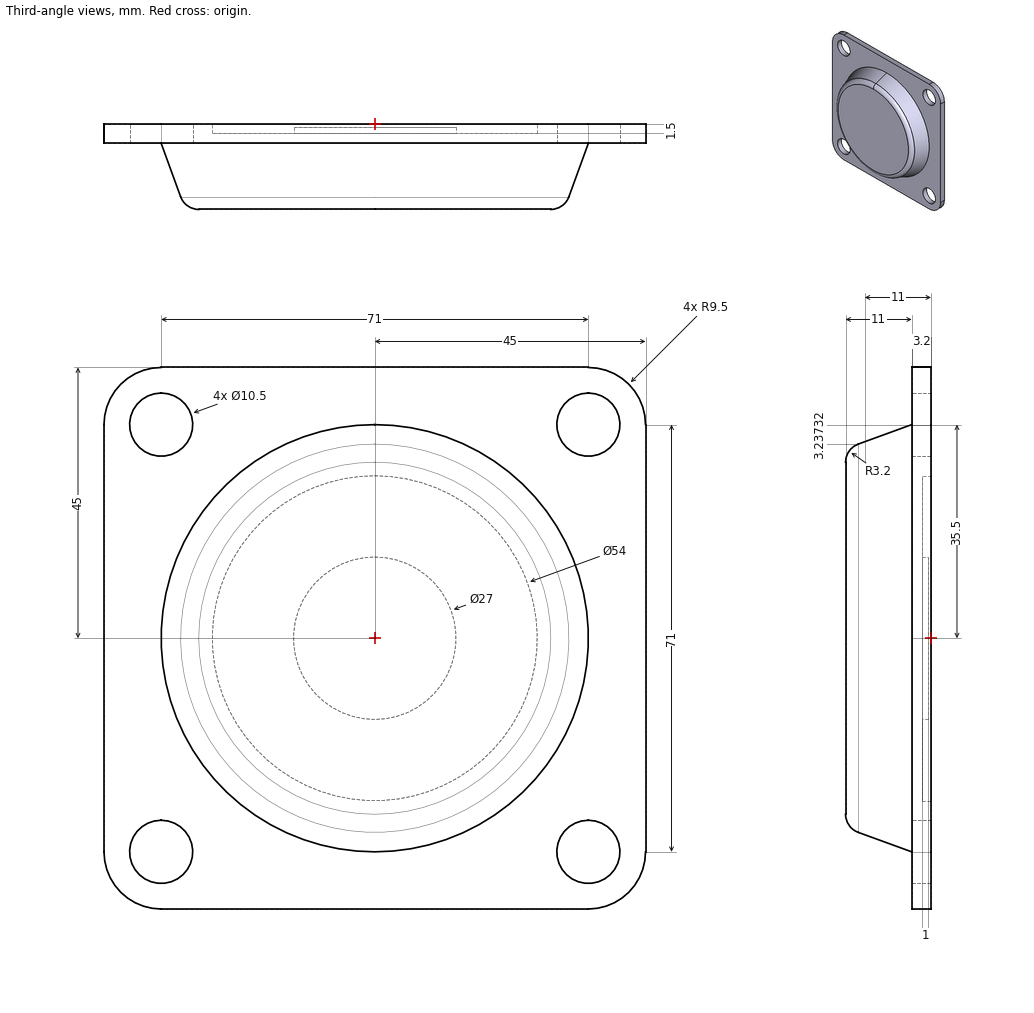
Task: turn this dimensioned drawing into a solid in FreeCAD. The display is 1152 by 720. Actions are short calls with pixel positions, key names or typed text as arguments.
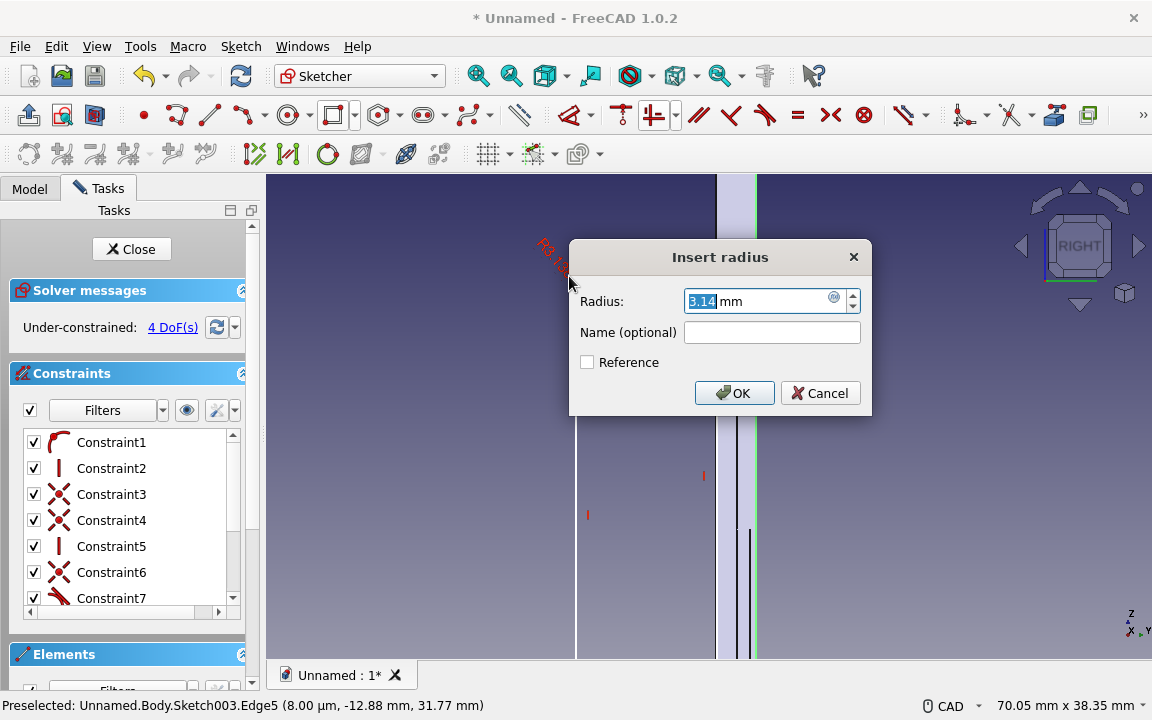
text(3.2)
key(Return)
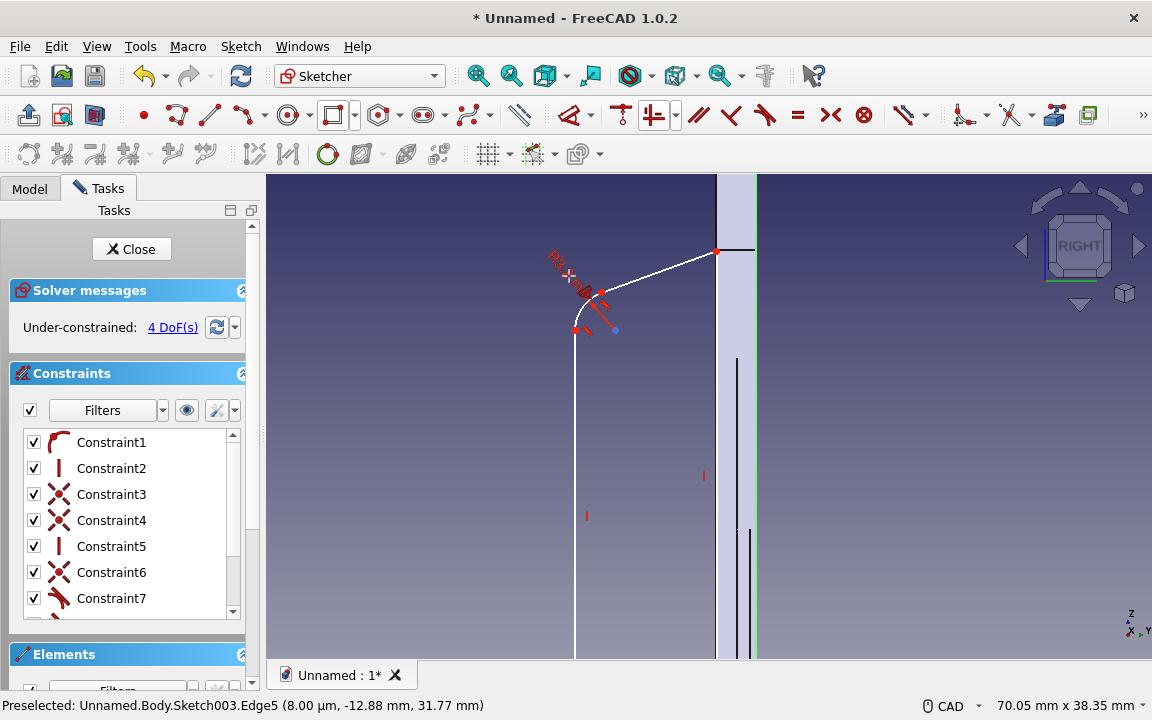
scroll(588, 298, down, 2)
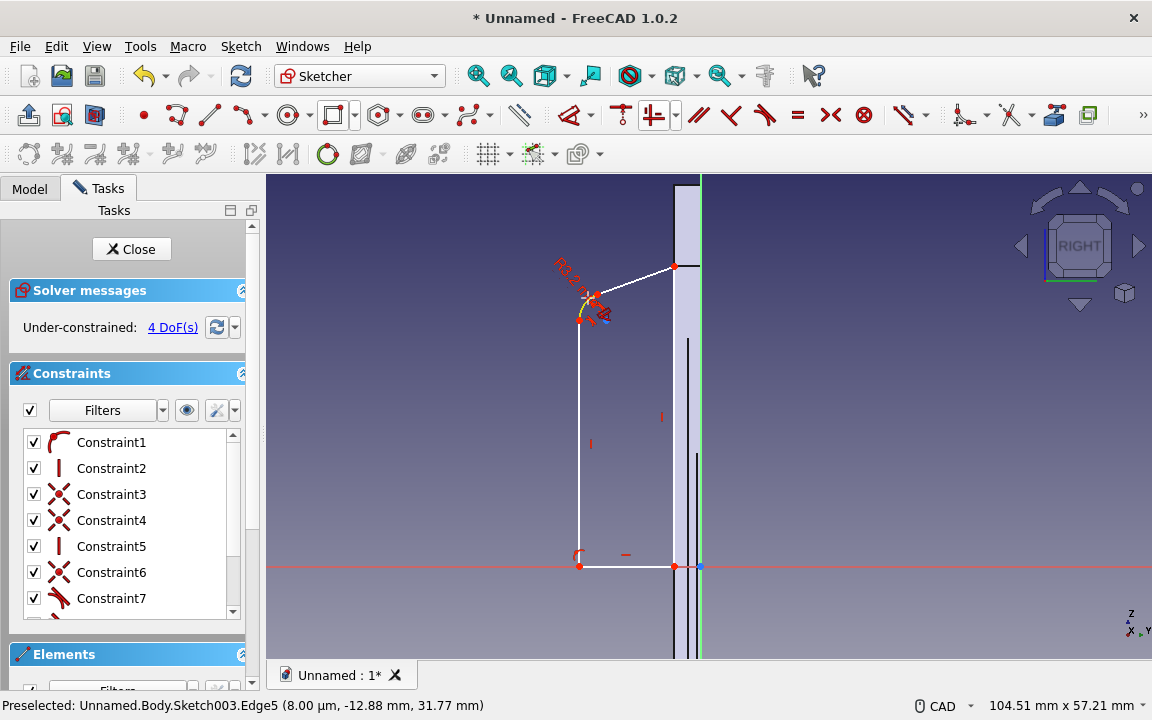
click(608, 567)
click(627, 601)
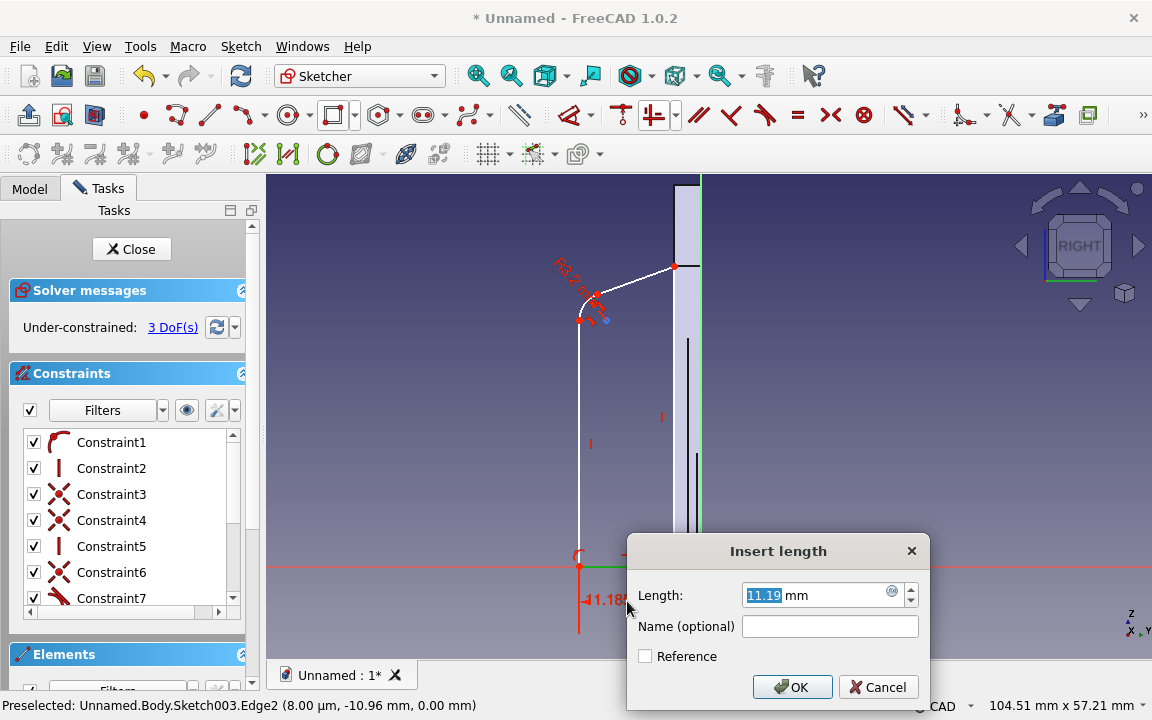
text(11)
key(Return)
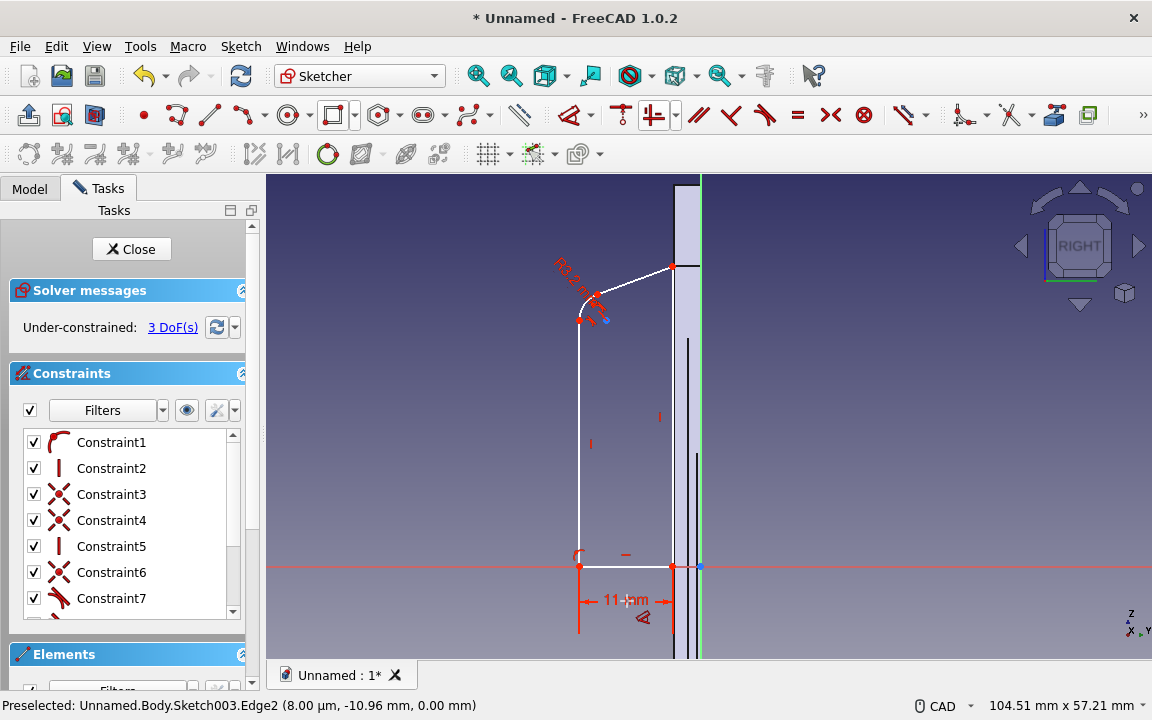
click(607, 320)
click(687, 286)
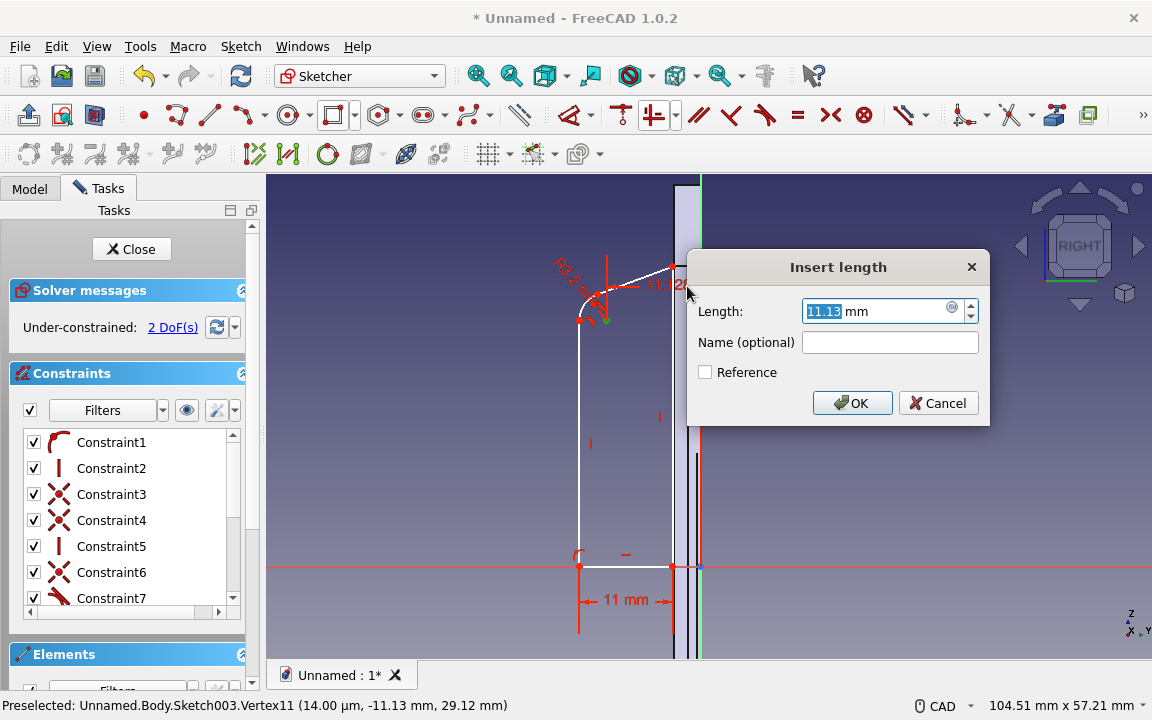
text(11)
key(Return)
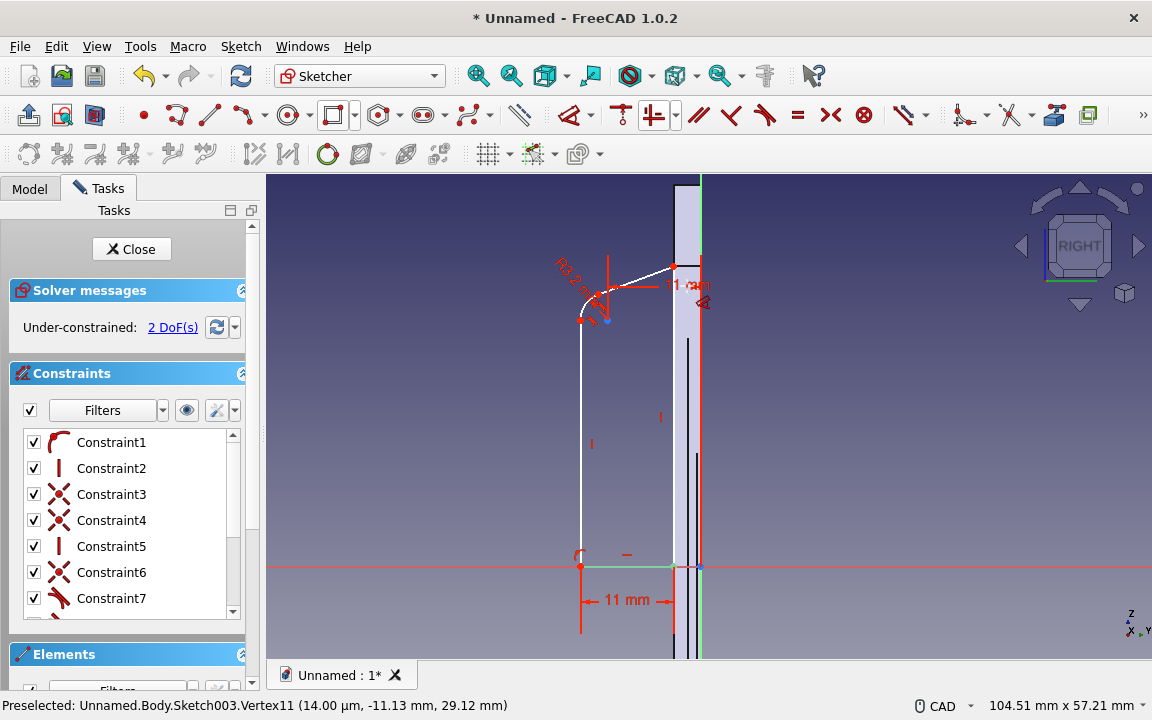
click(674, 477)
click(640, 417)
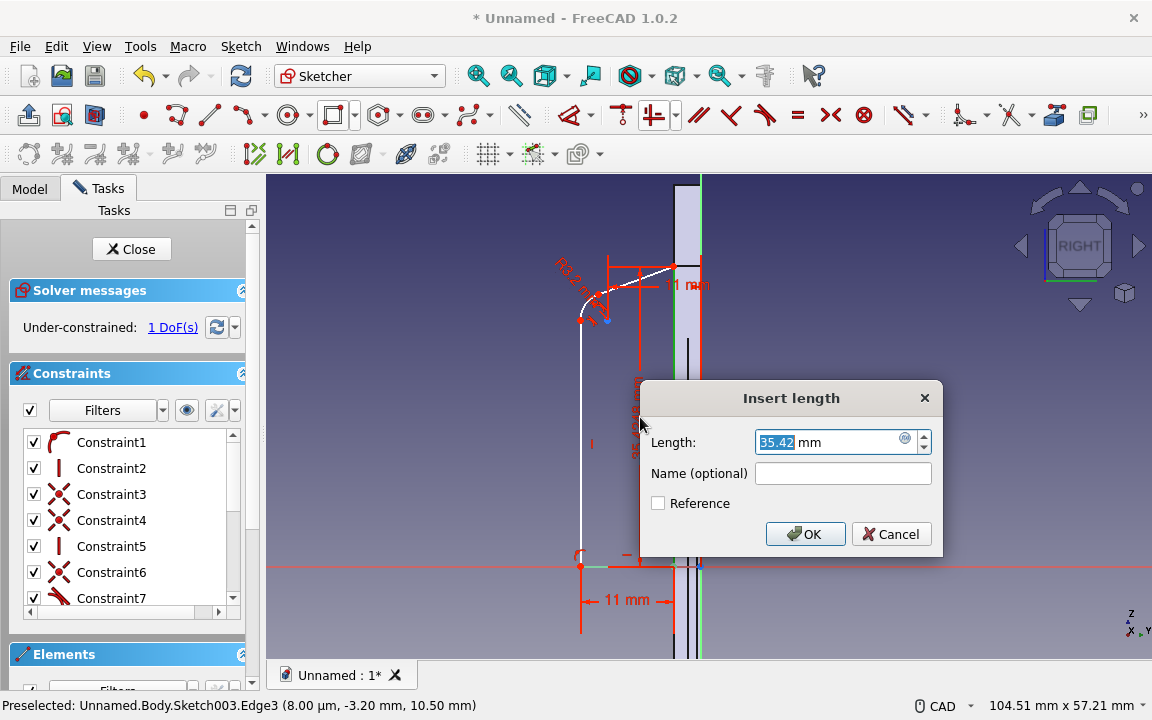
text(35.5)
key(Return)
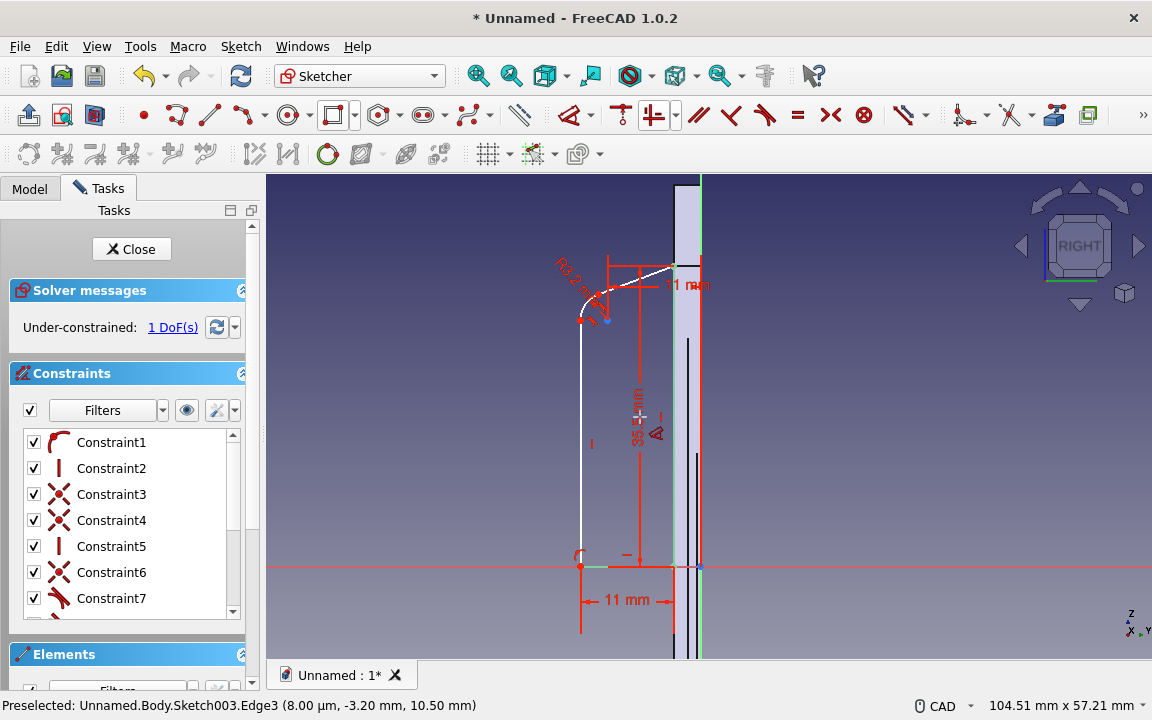
scroll(651, 275, up, 2)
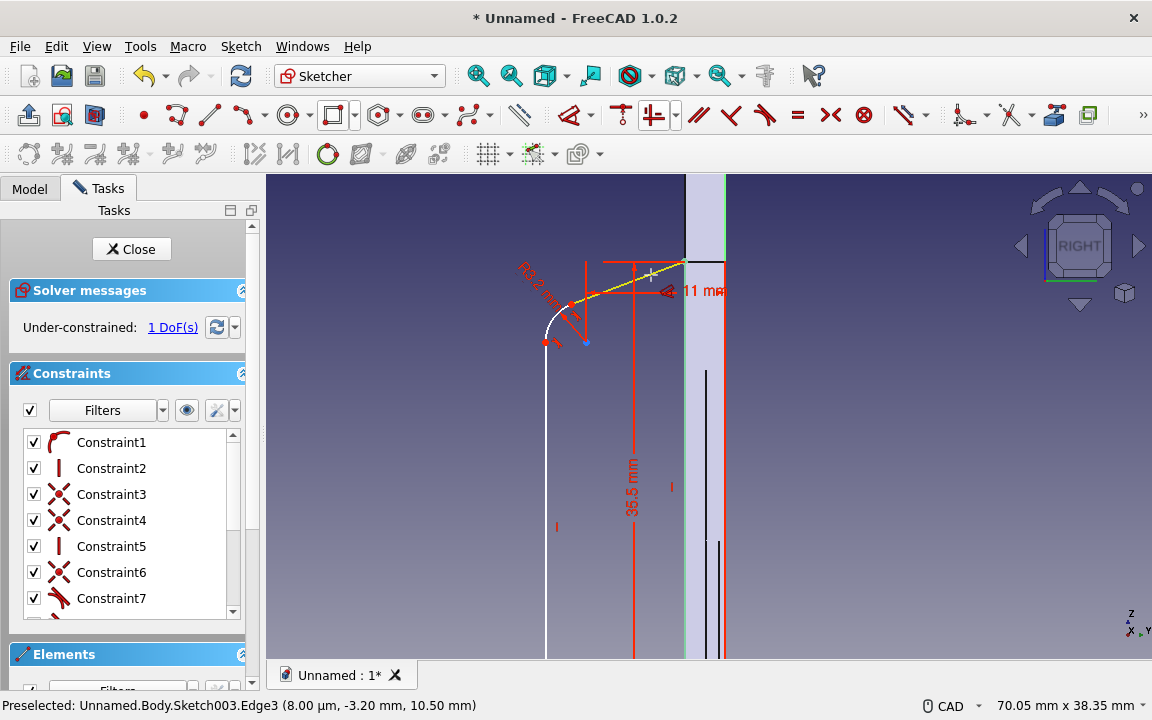
click(651, 274)
click(743, 268)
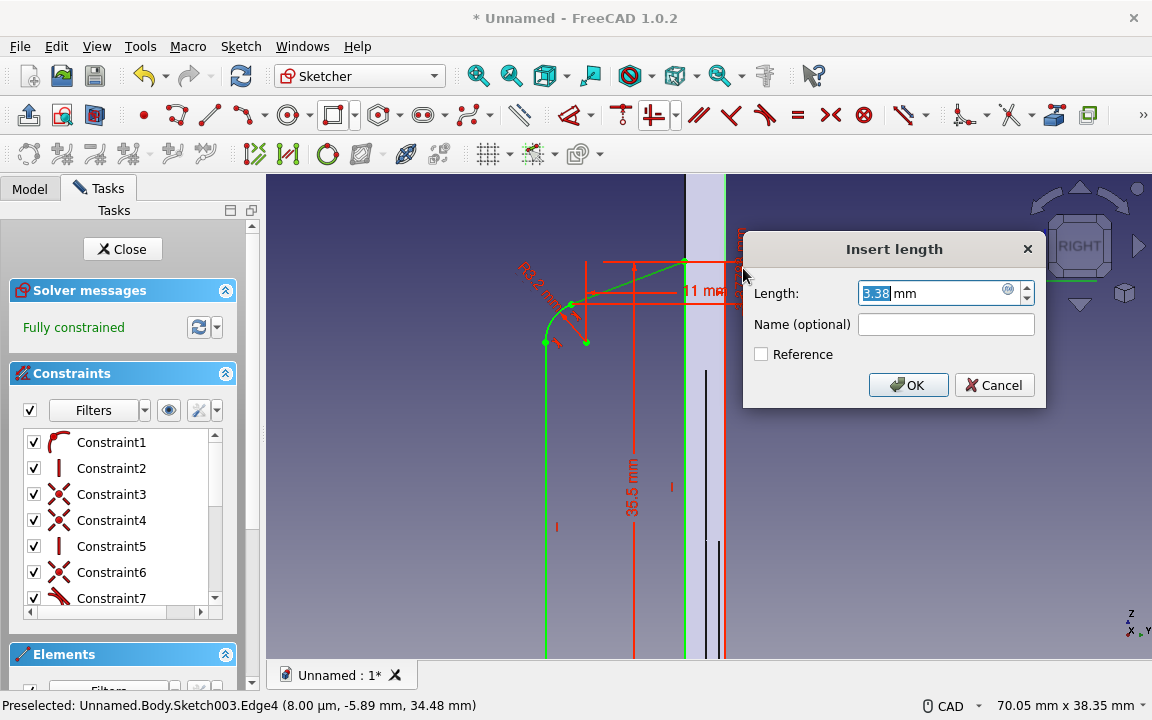
text(3.23732)
key(Return)
key(Escape)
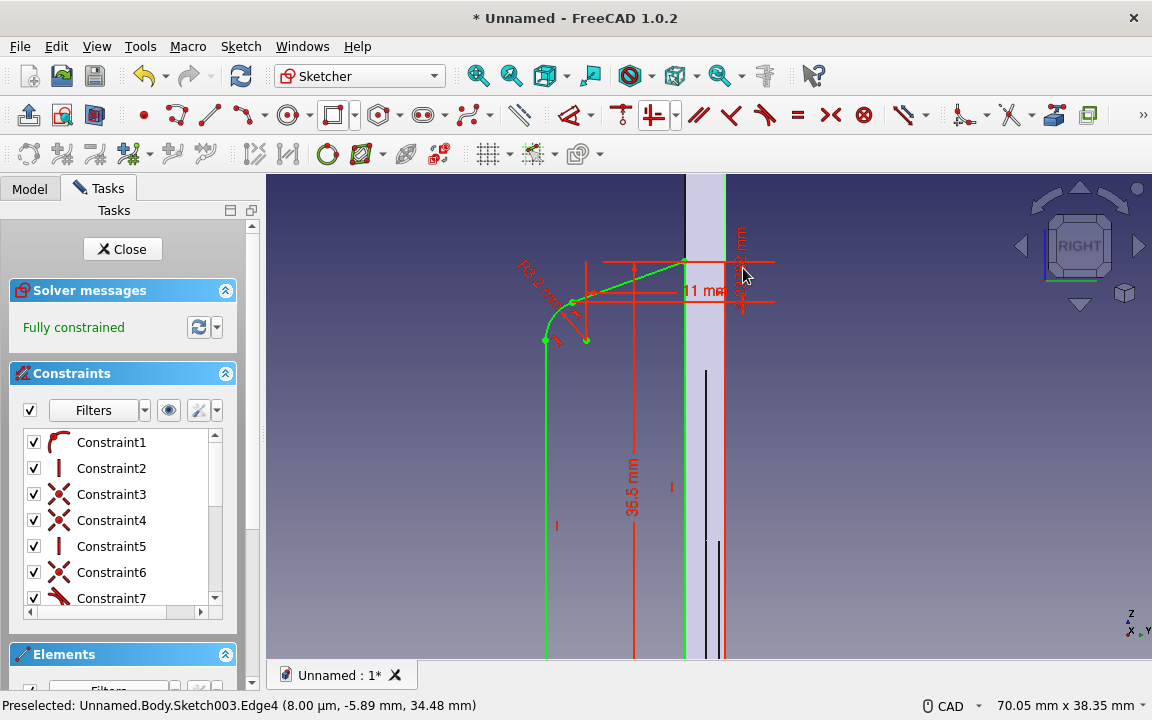
click(123, 249)